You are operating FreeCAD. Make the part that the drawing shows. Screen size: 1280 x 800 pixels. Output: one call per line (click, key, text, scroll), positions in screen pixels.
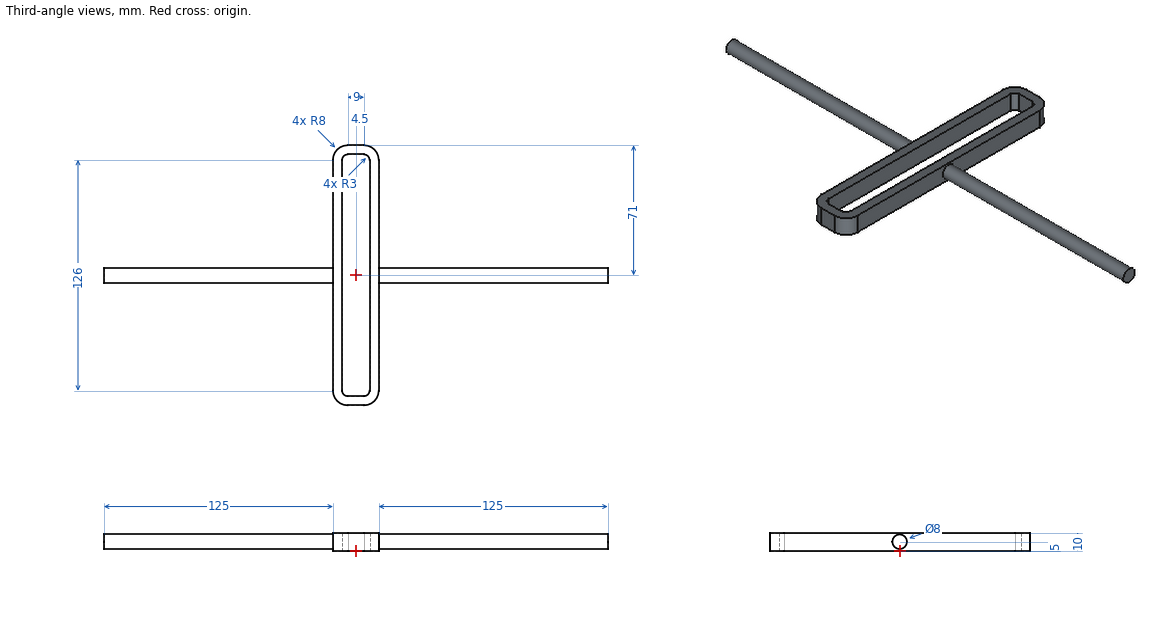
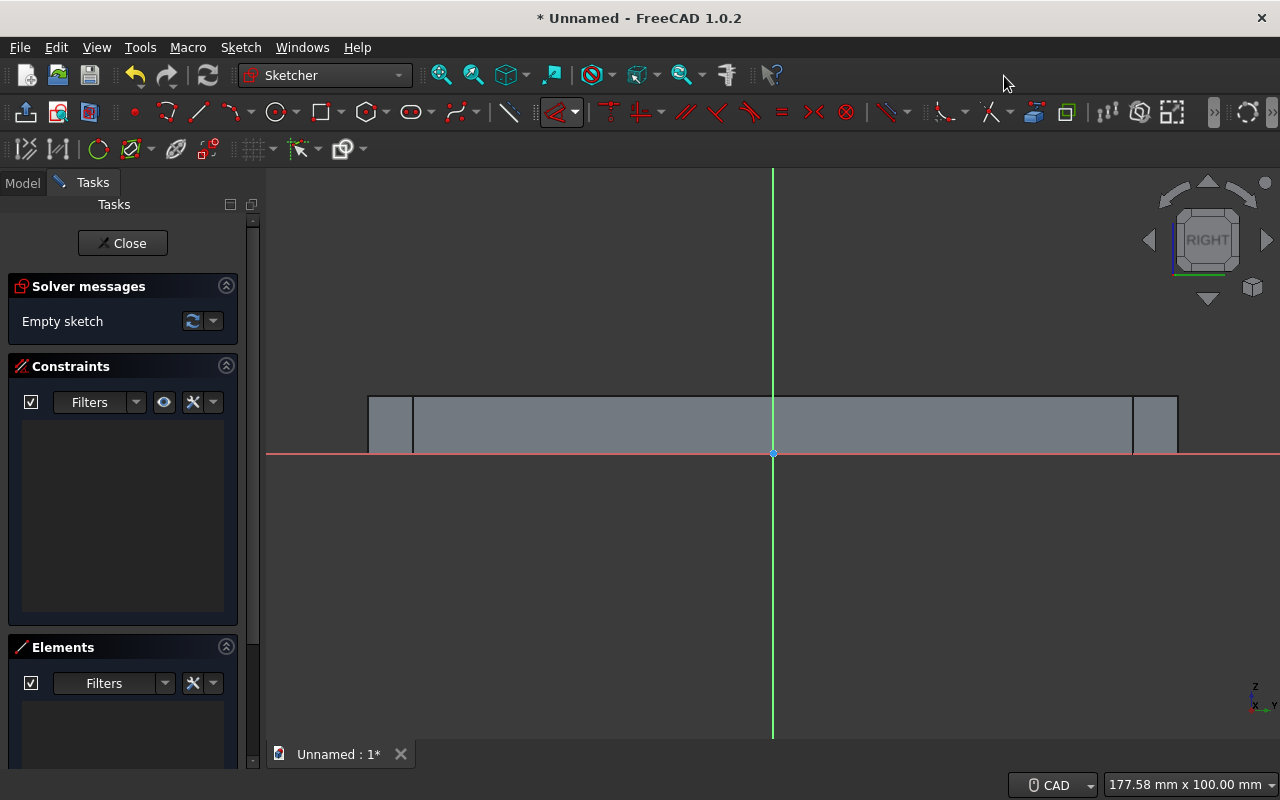
scroll(784, 424, up, 10)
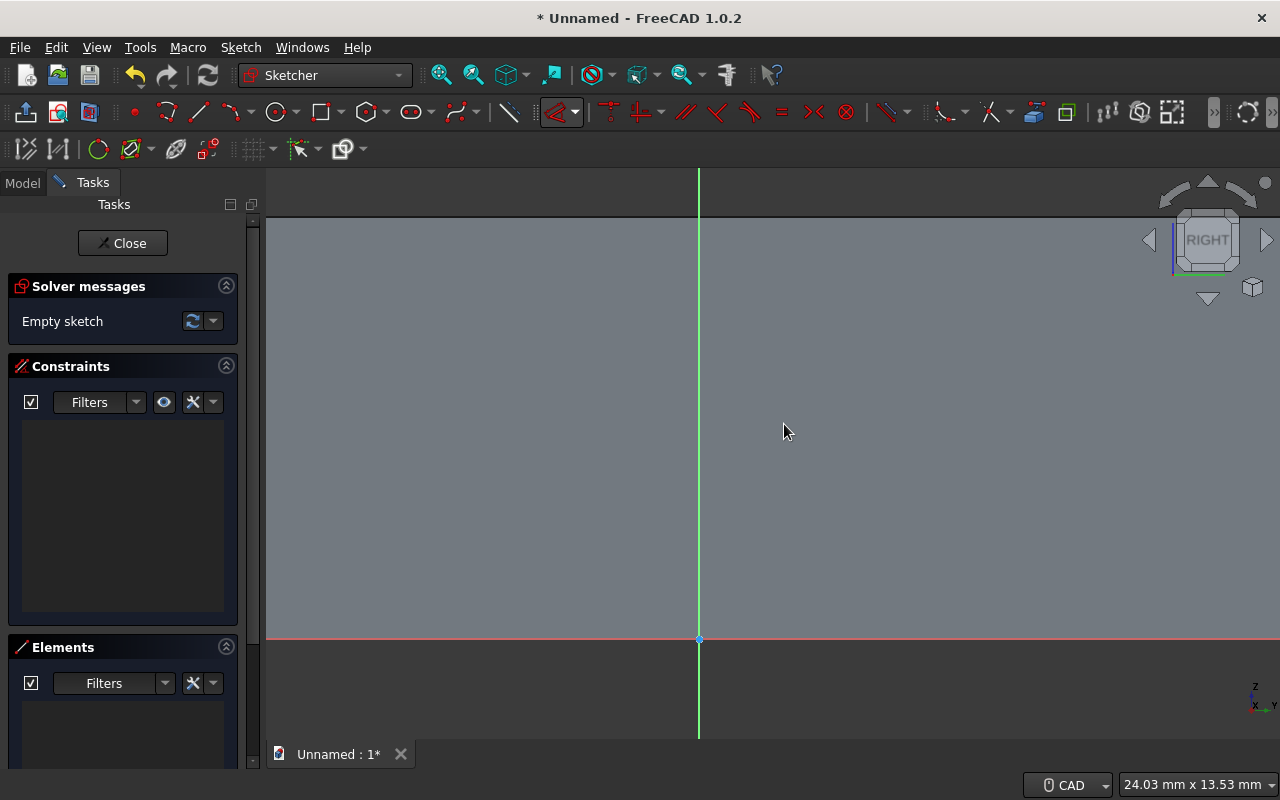
click(276, 112)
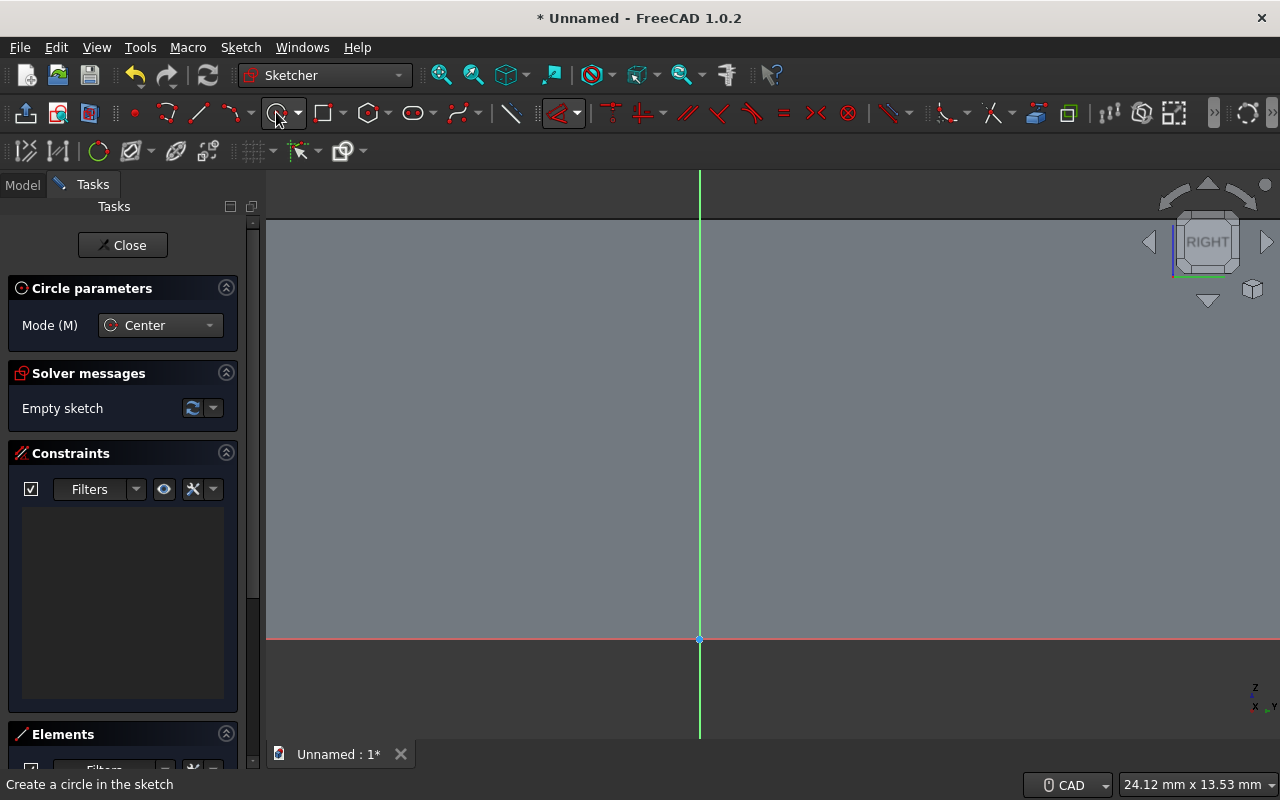
click(700, 429)
click(819, 310)
key(Escape)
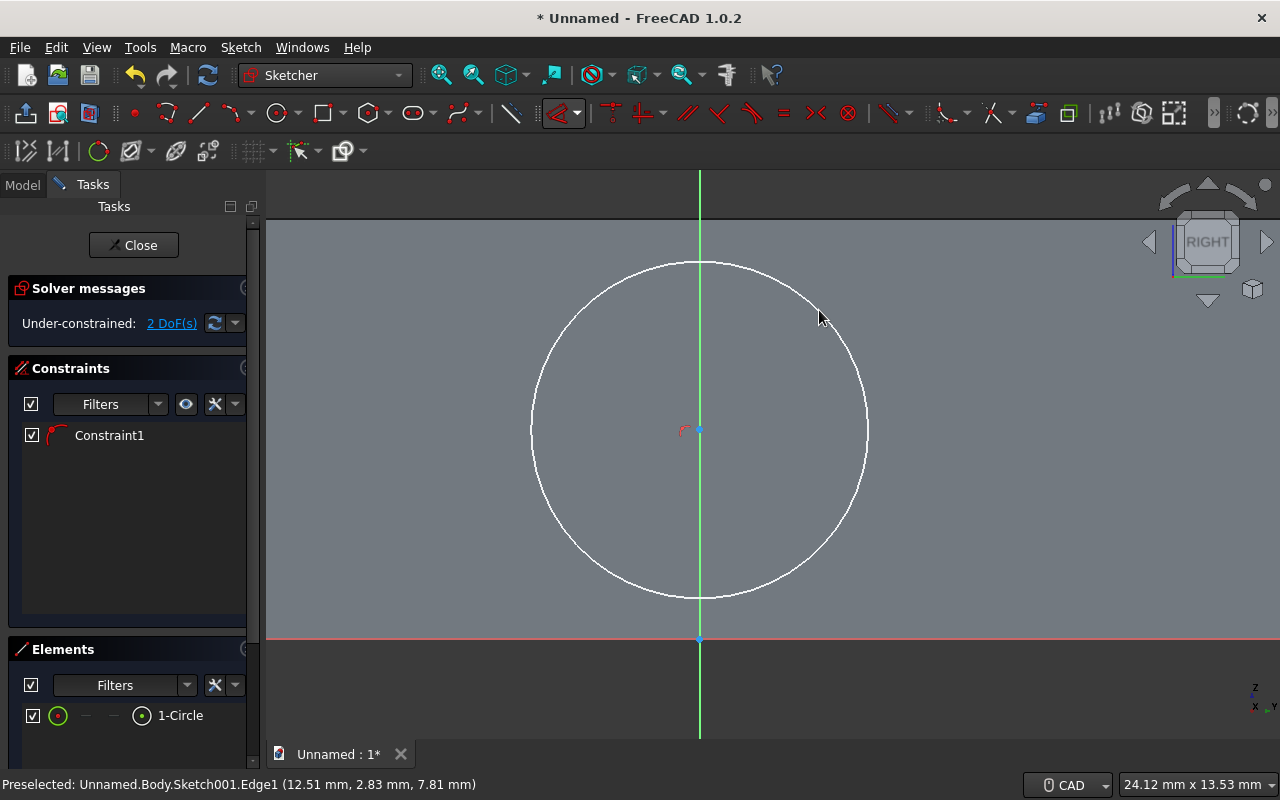
click(818, 310)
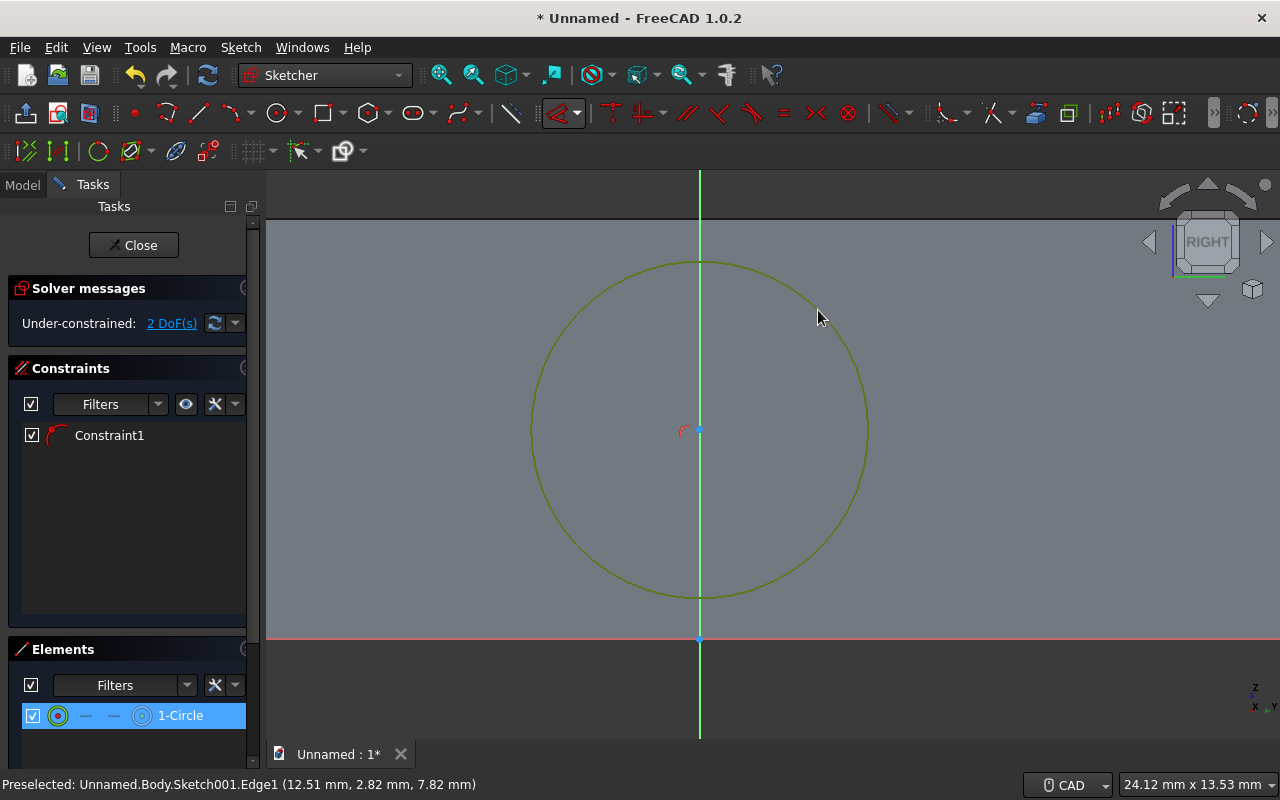
click(580, 114)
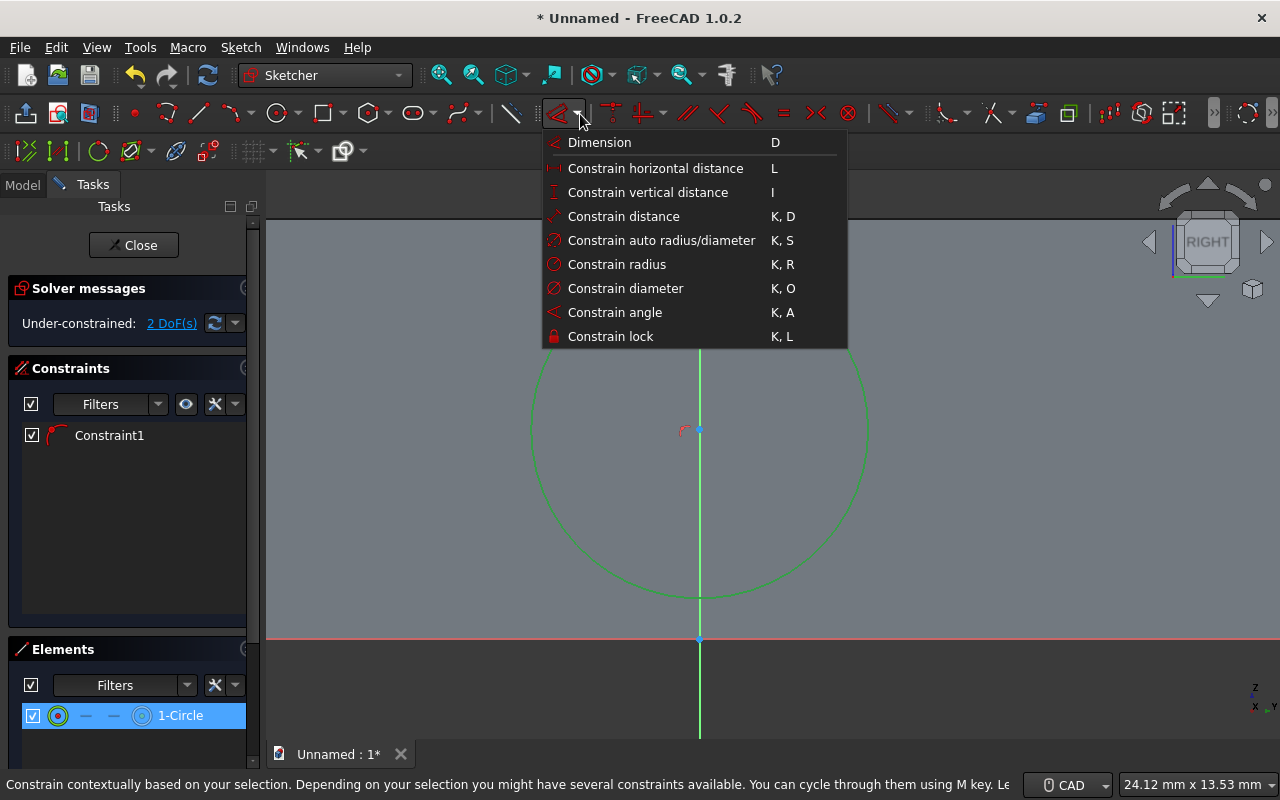
click(695, 288)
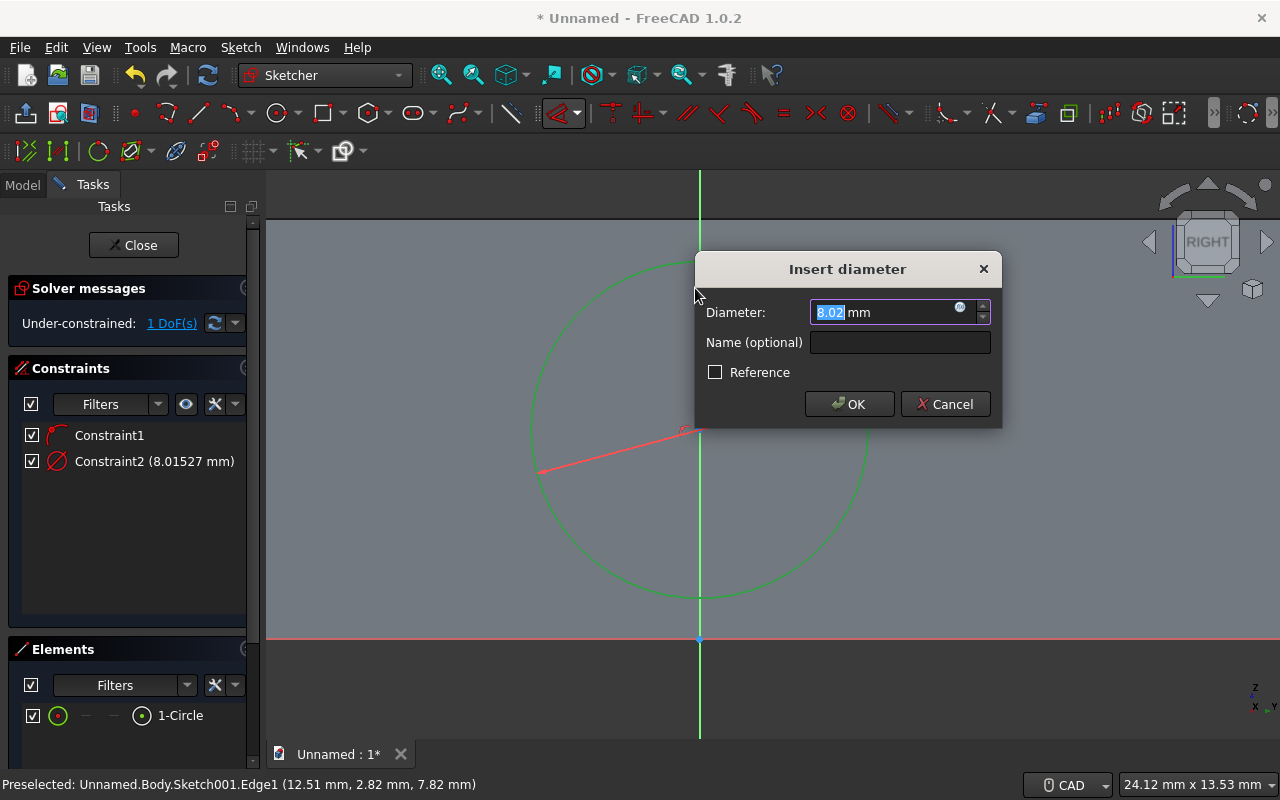
text(8)
key(Return)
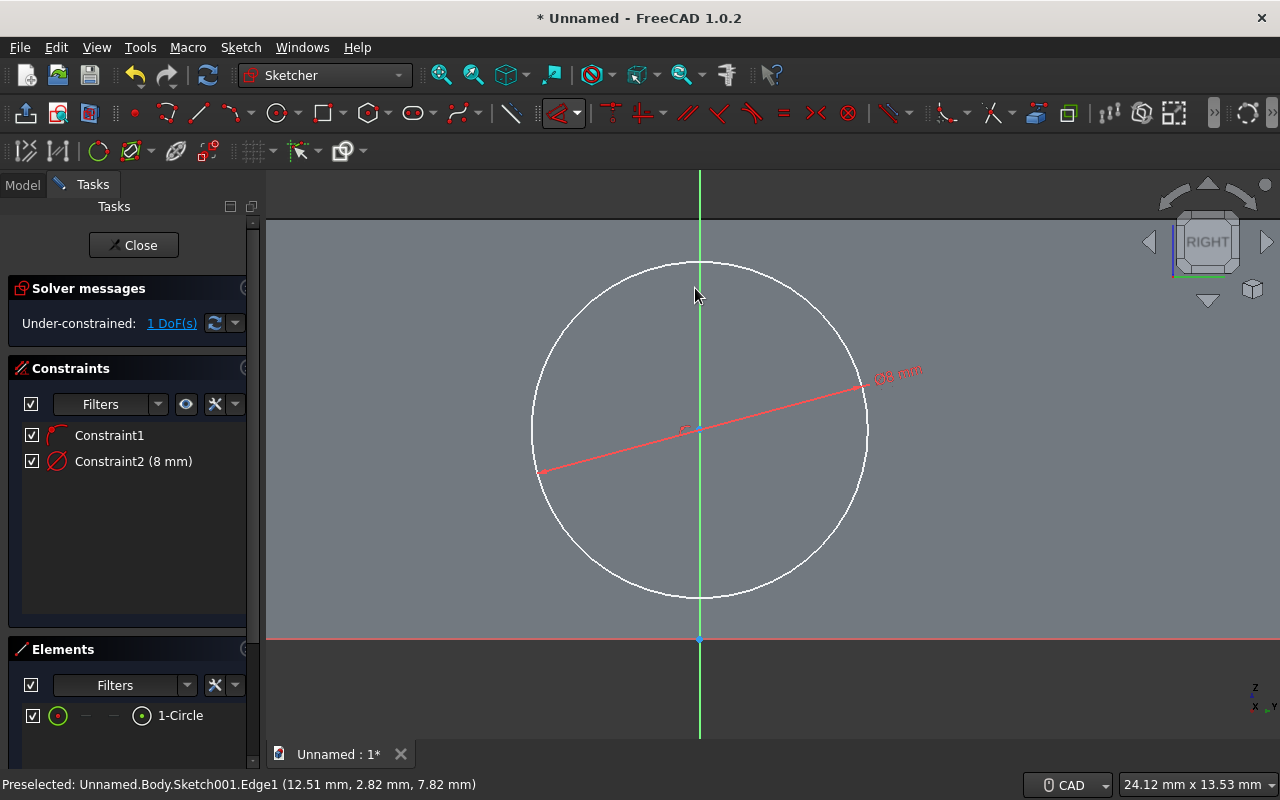
click(700, 430)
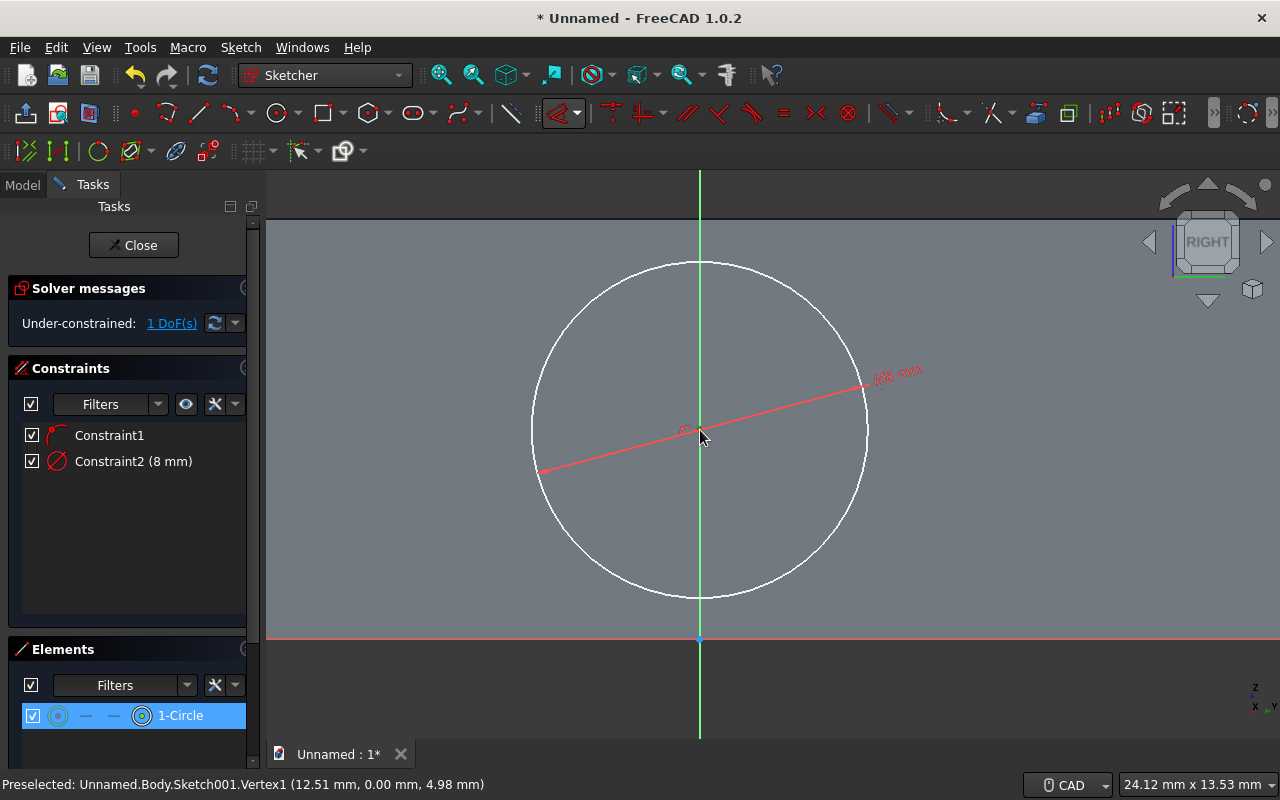
click(580, 114)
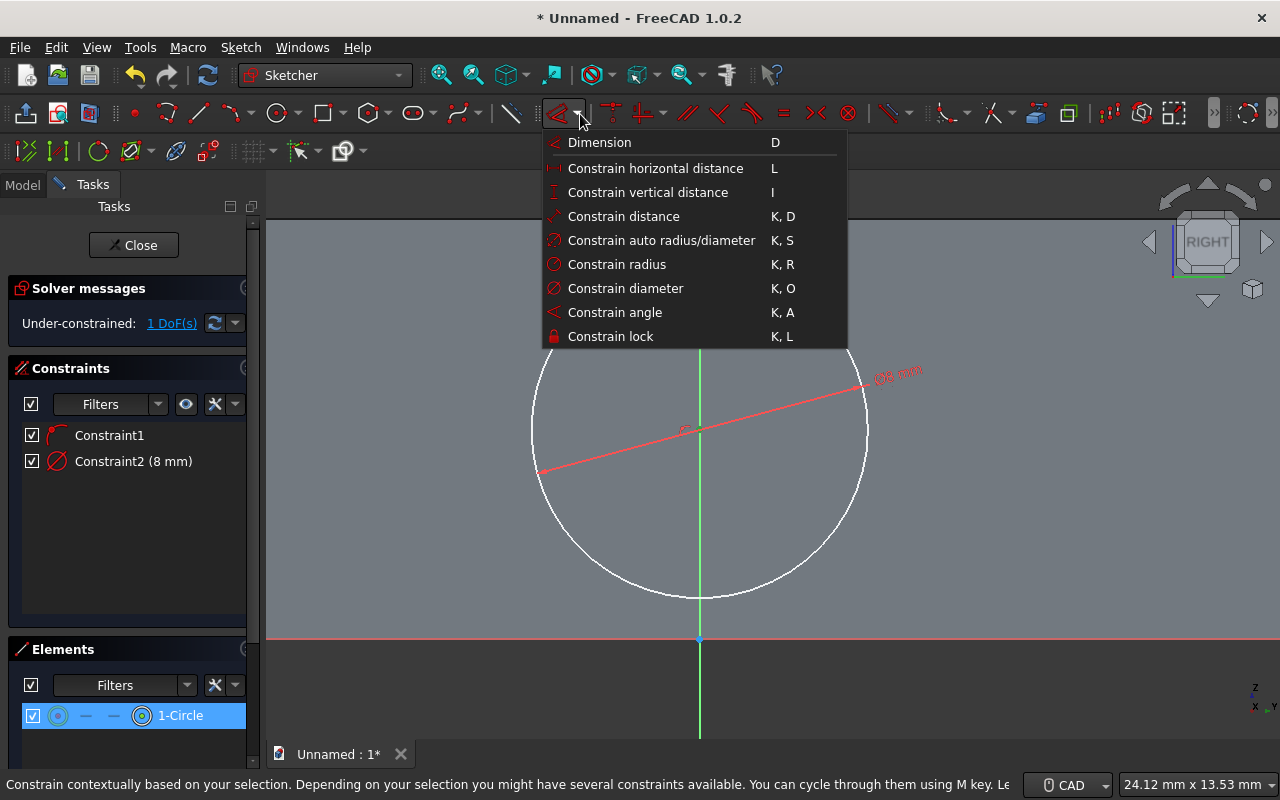
click(695, 192)